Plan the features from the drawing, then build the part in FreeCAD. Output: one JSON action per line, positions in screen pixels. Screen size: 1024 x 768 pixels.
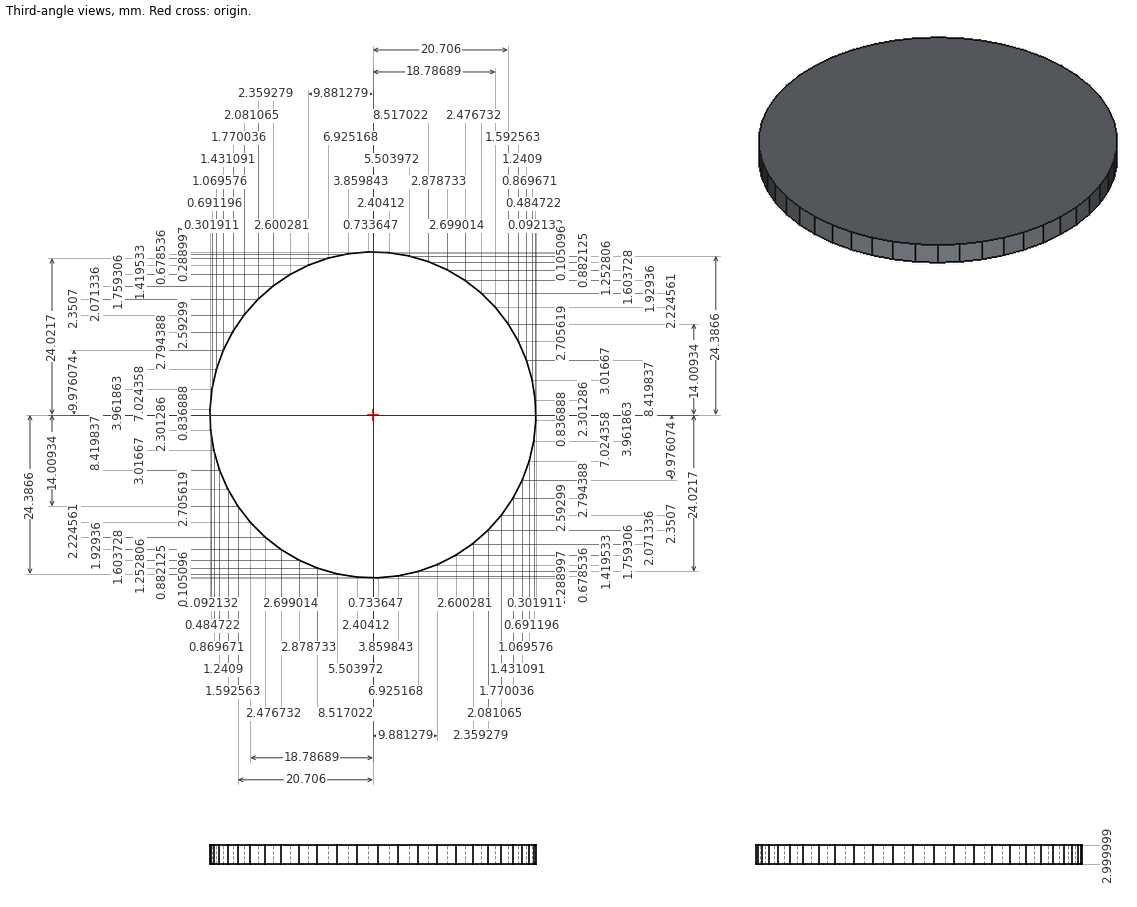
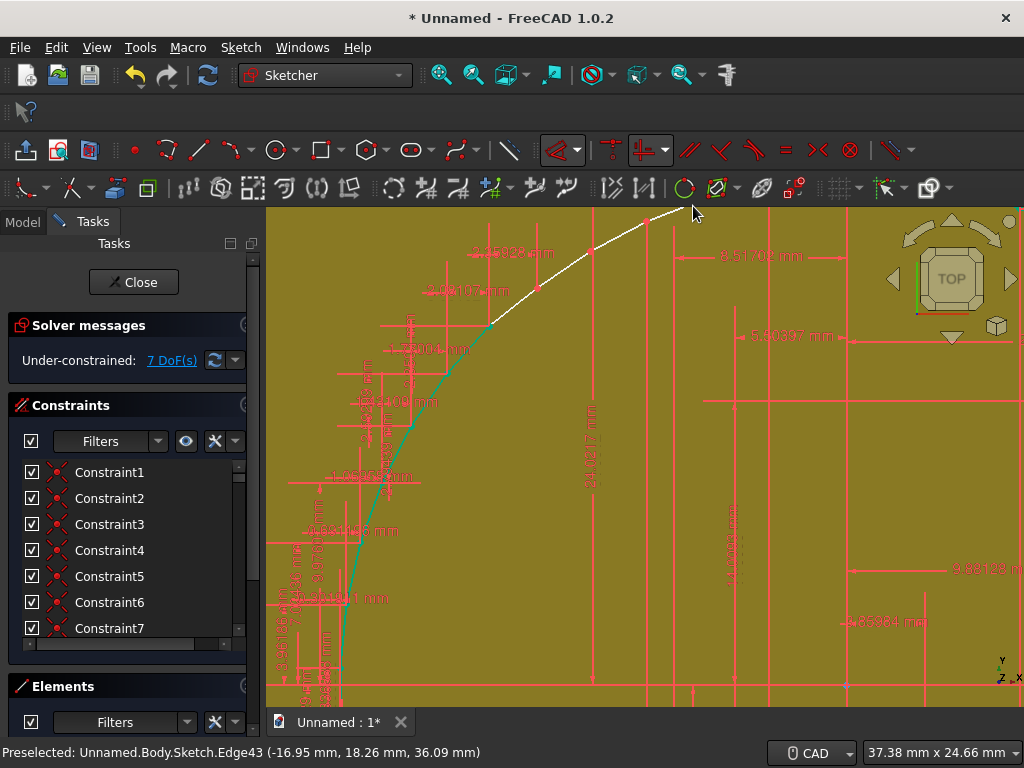
{"action": "left_click", "coordinate": [504, 315]}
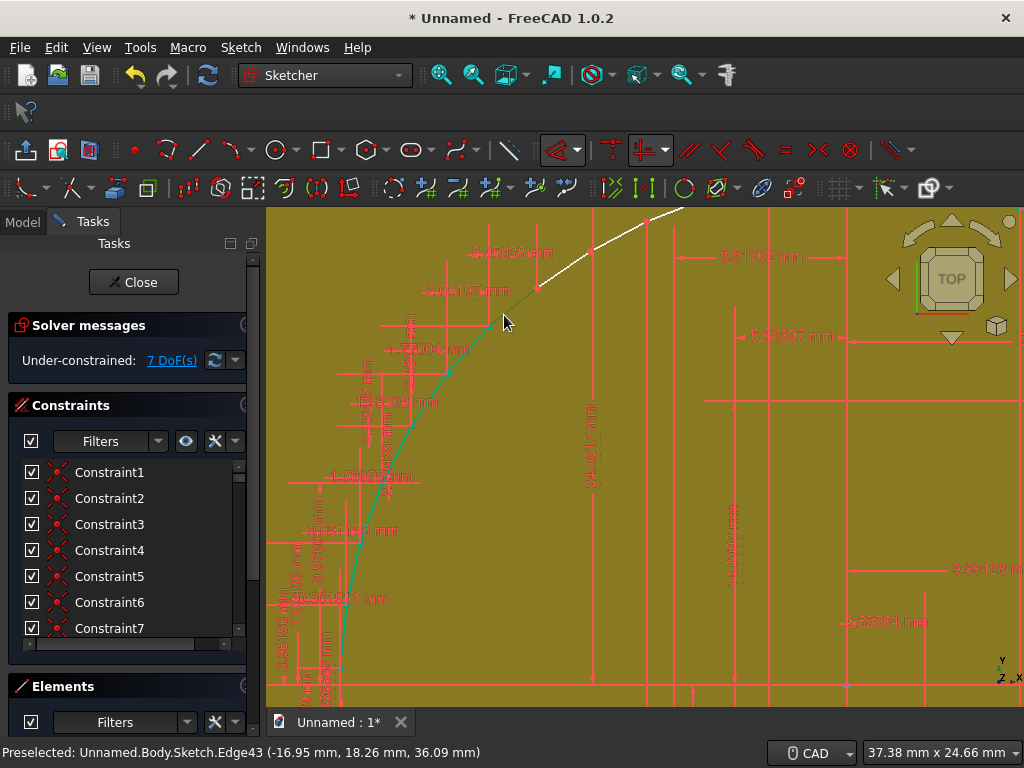
{"action": "left_click", "coordinate": [580, 150]}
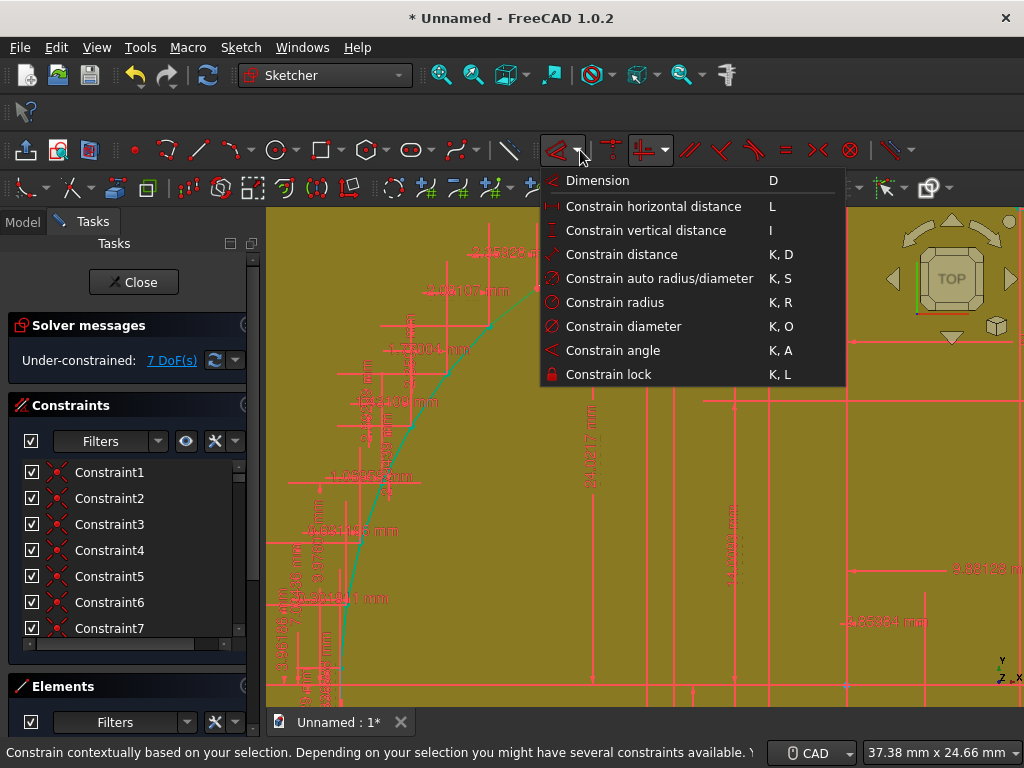
{"action": "left_click", "coordinate": [693, 230]}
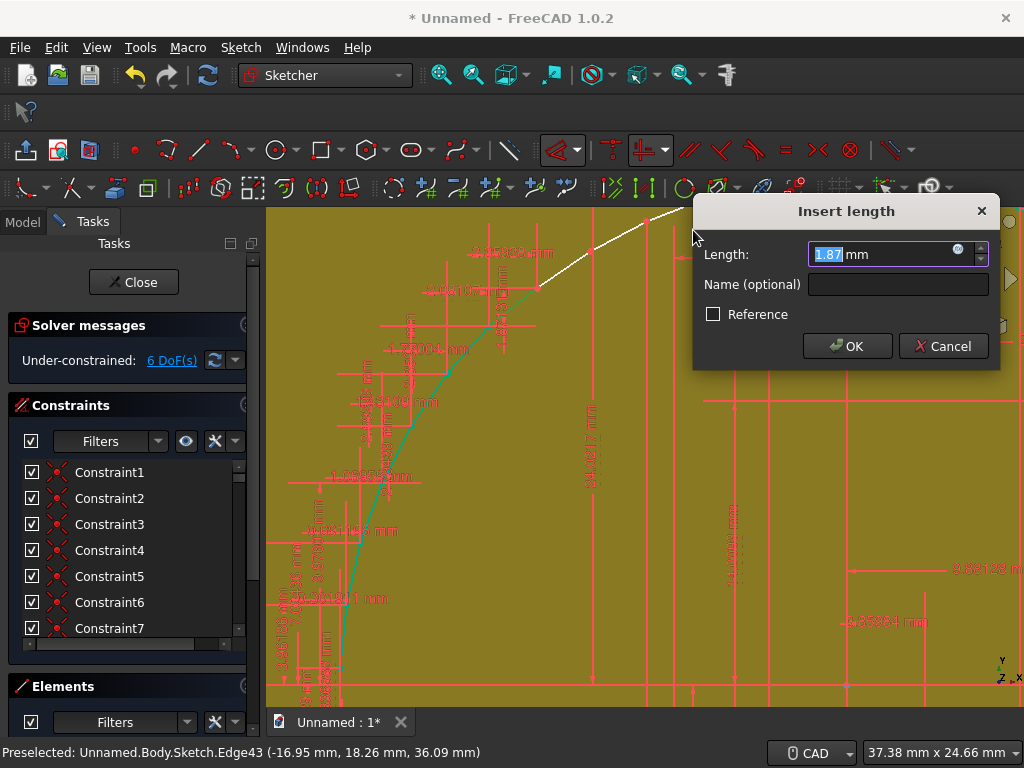
{"action": "type", "text": "2.071336"}
{"action": "key", "text": "Return"}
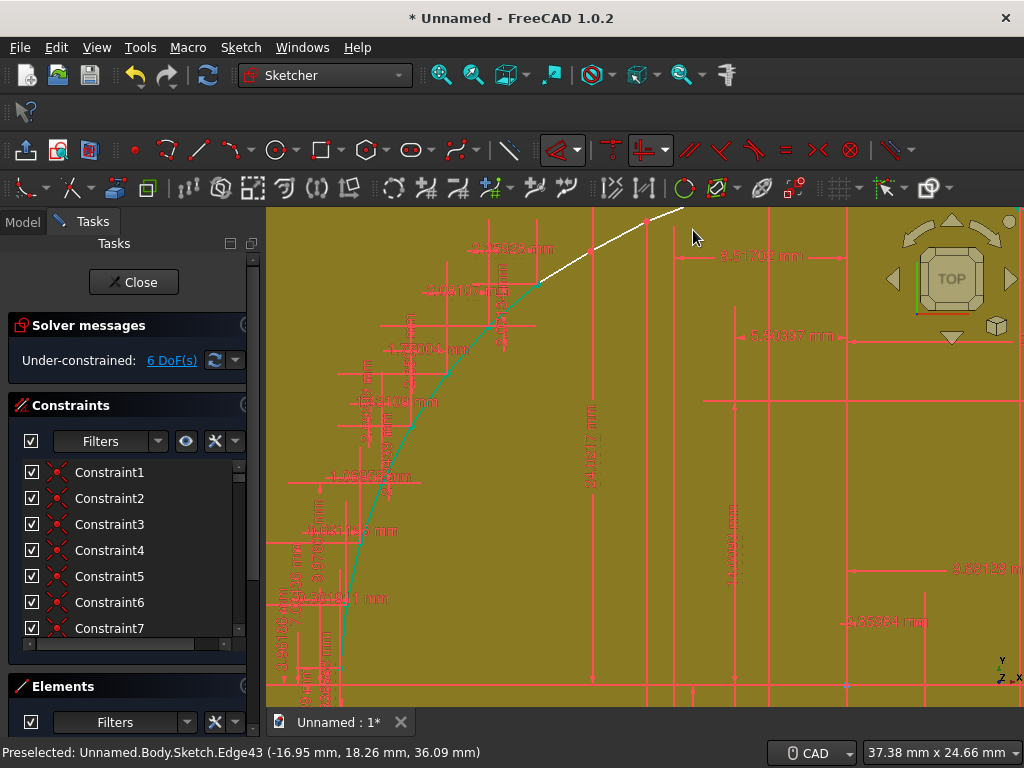
{"action": "left_click", "coordinate": [553, 274]}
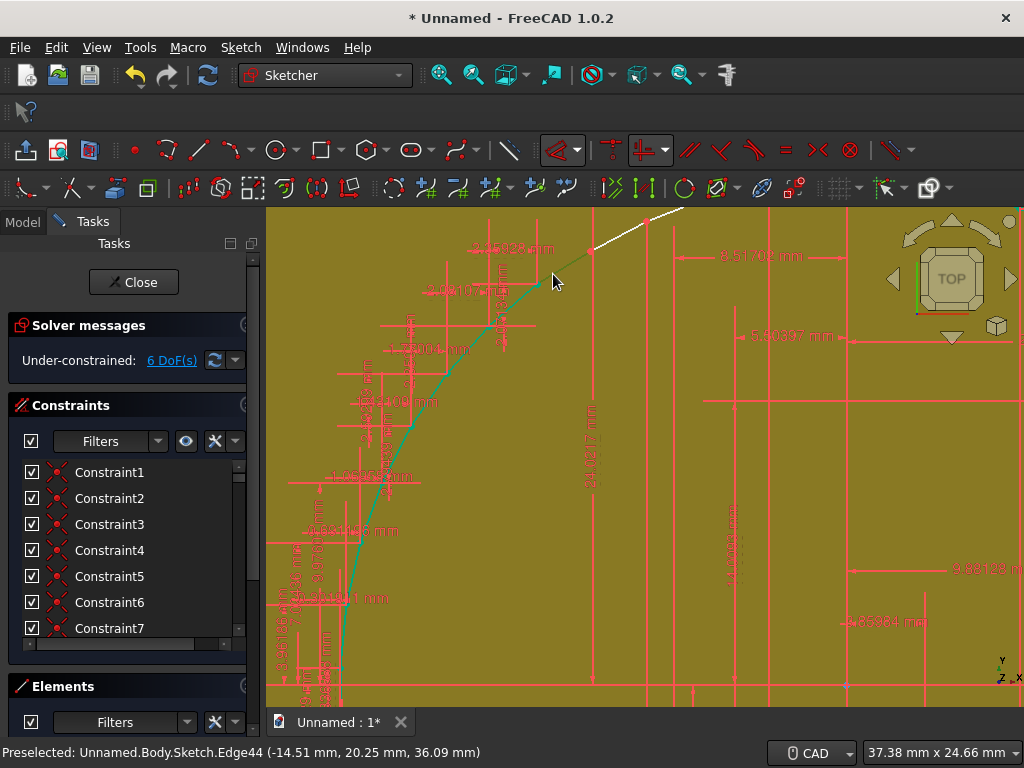
{"action": "left_click", "coordinate": [580, 150]}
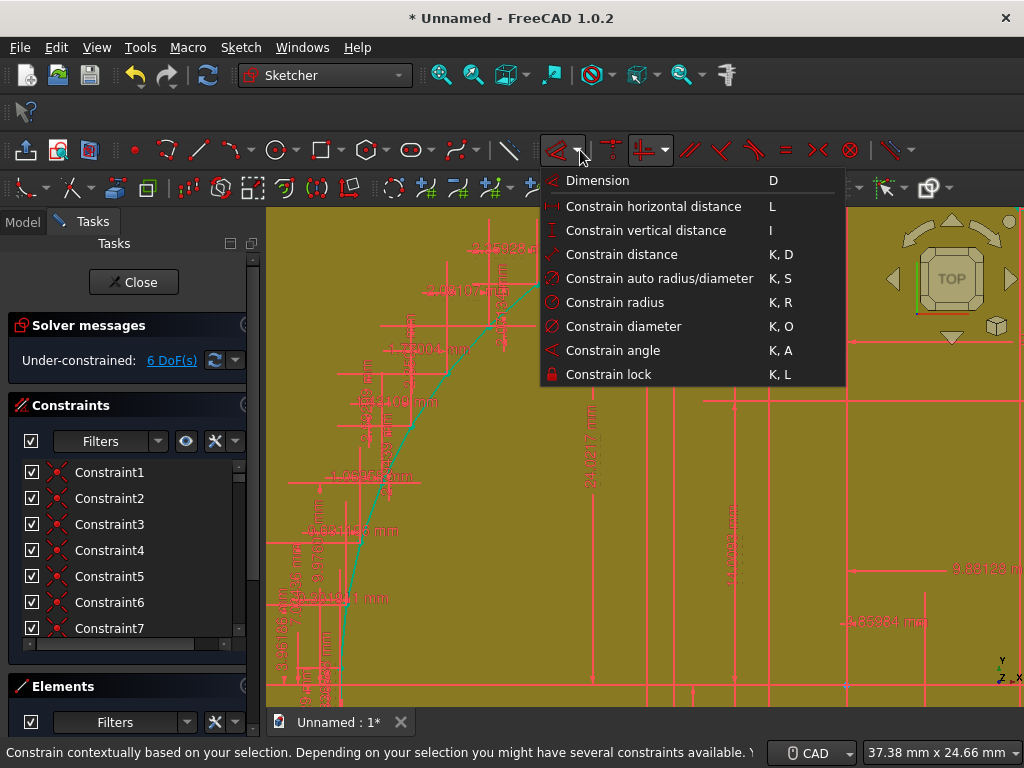
{"action": "left_click", "coordinate": [693, 206]}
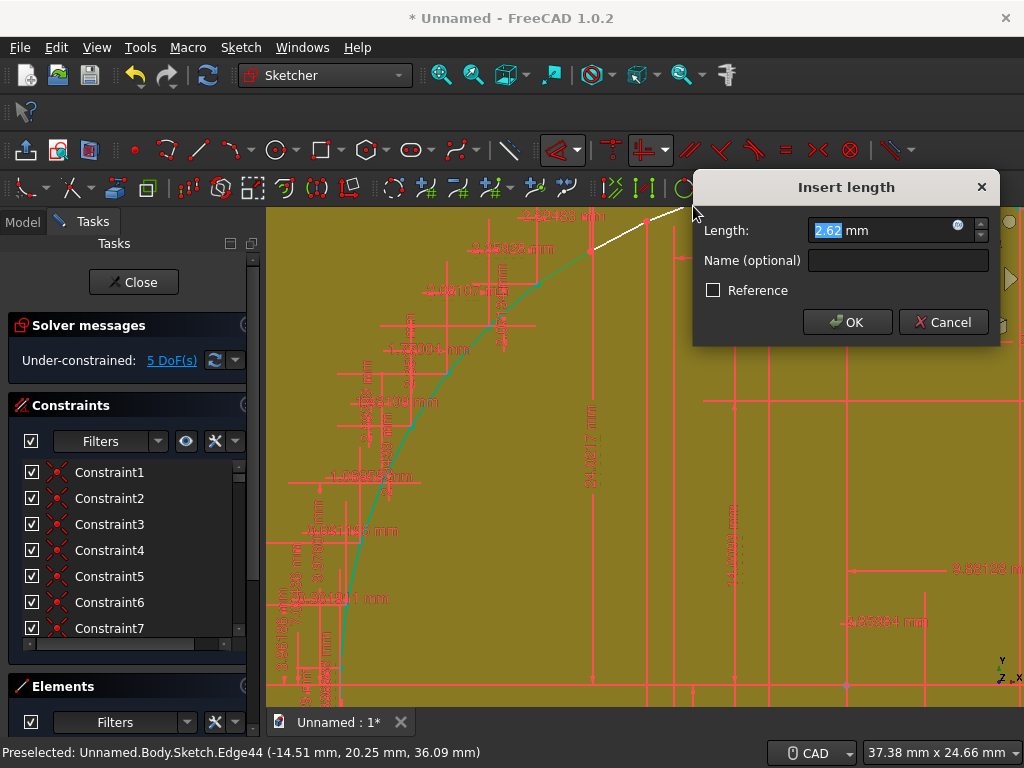
{"action": "type", "text": "2.600281"}
{"action": "key", "text": "Return"}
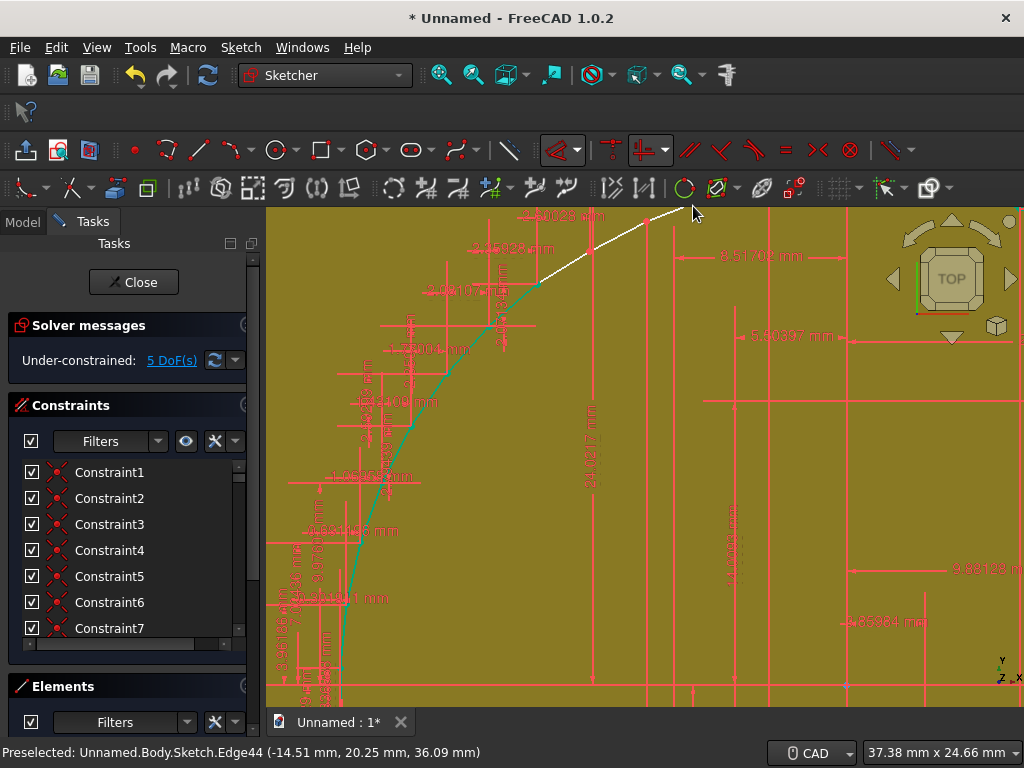
{"action": "left_click", "coordinate": [553, 274]}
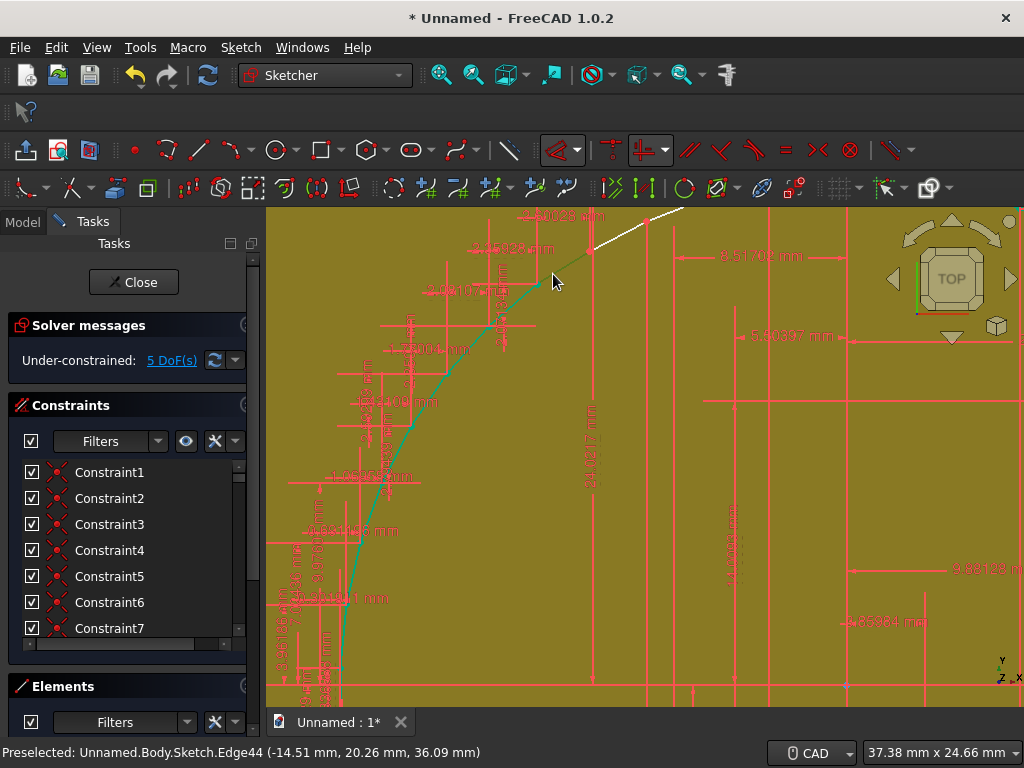
{"action": "left_click", "coordinate": [580, 150]}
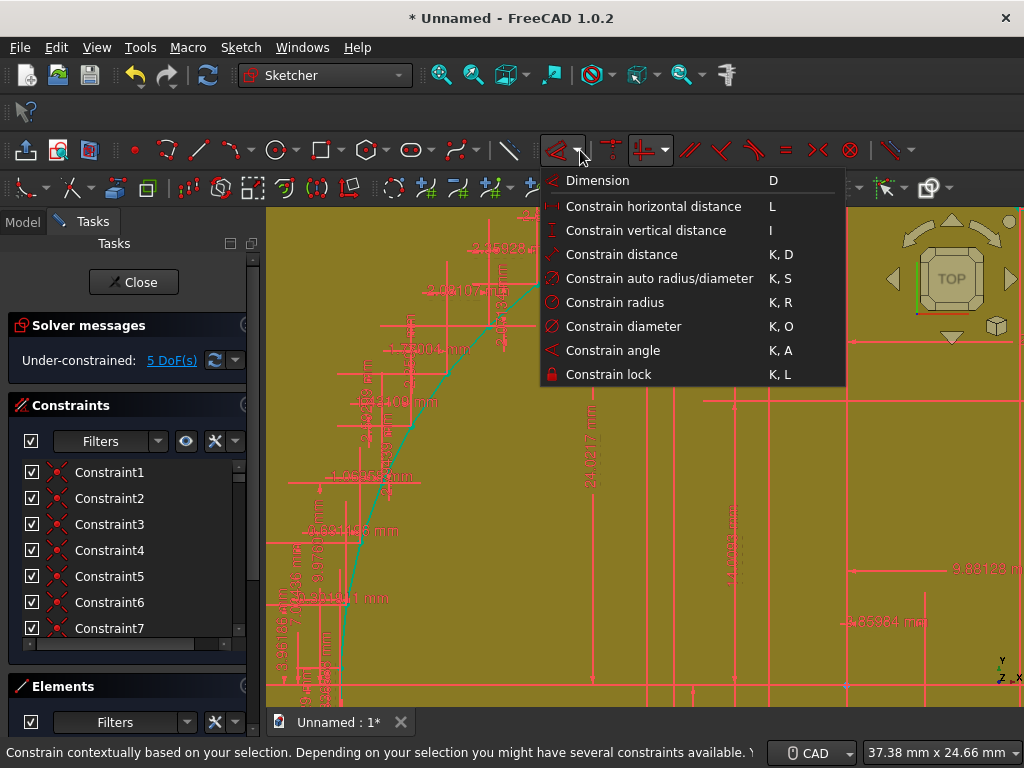
{"action": "left_click", "coordinate": [693, 230]}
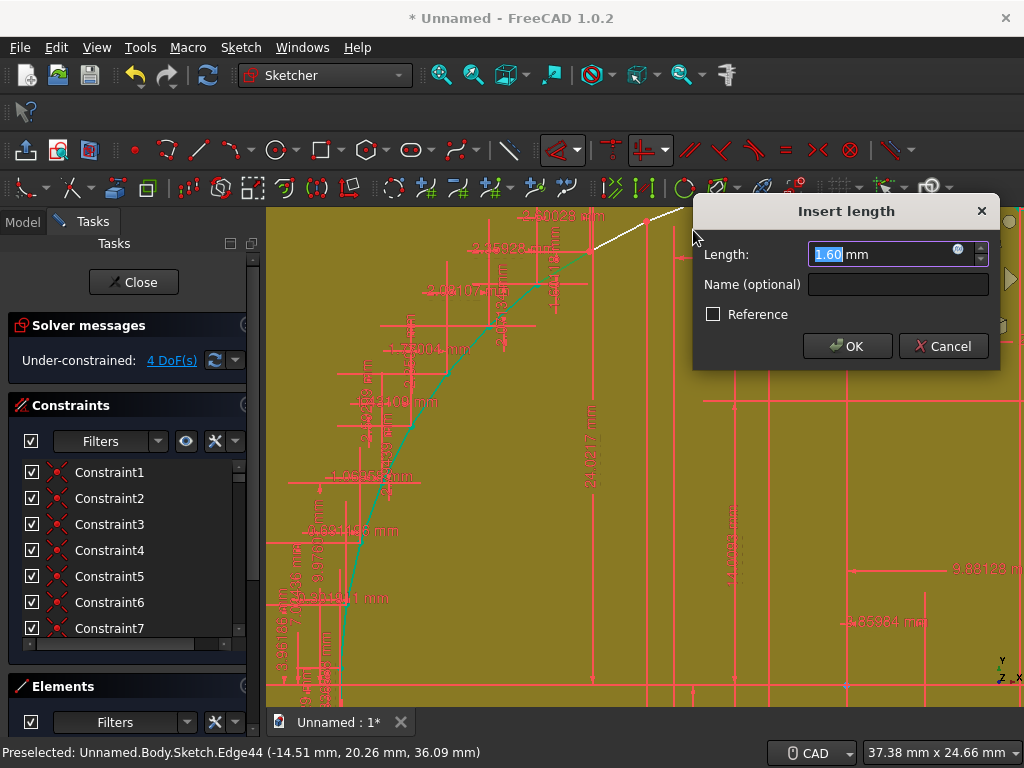
{"action": "type", "text": "1.759306"}
{"action": "key", "text": "Return"}